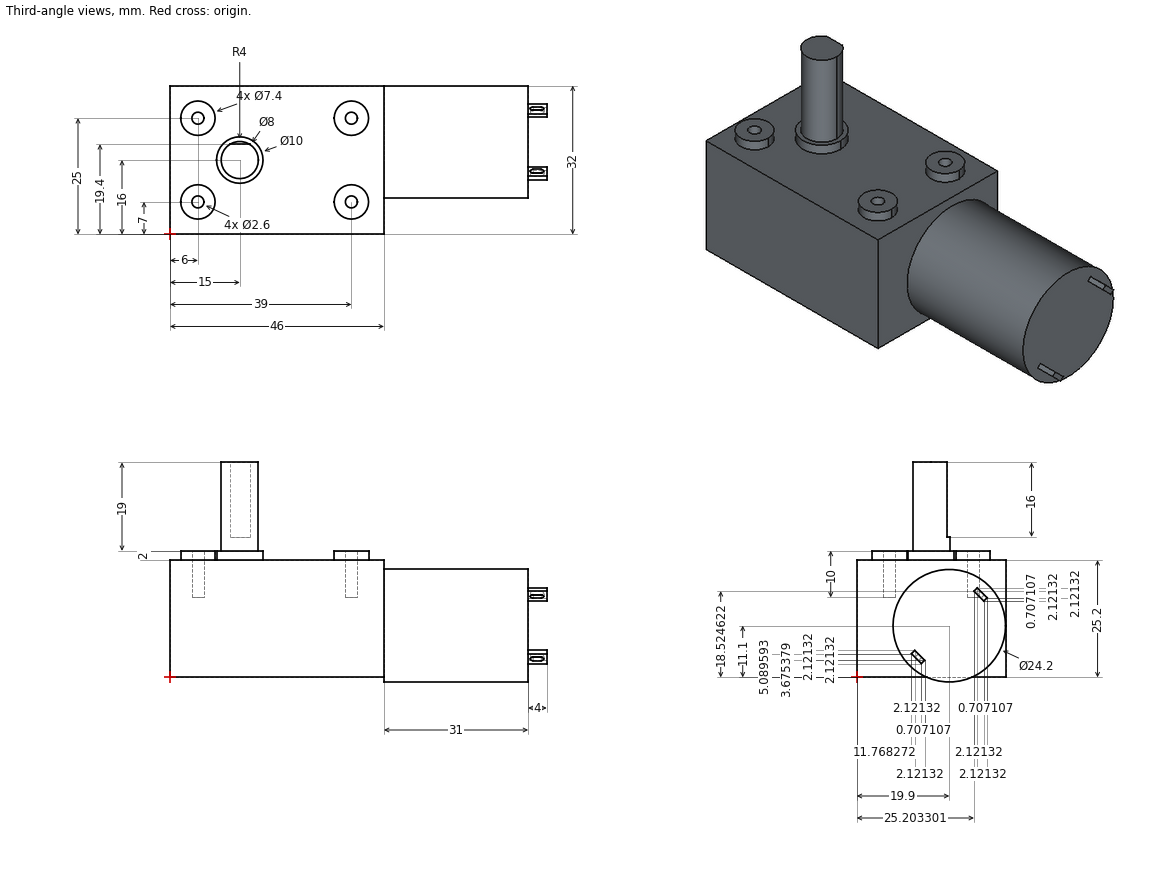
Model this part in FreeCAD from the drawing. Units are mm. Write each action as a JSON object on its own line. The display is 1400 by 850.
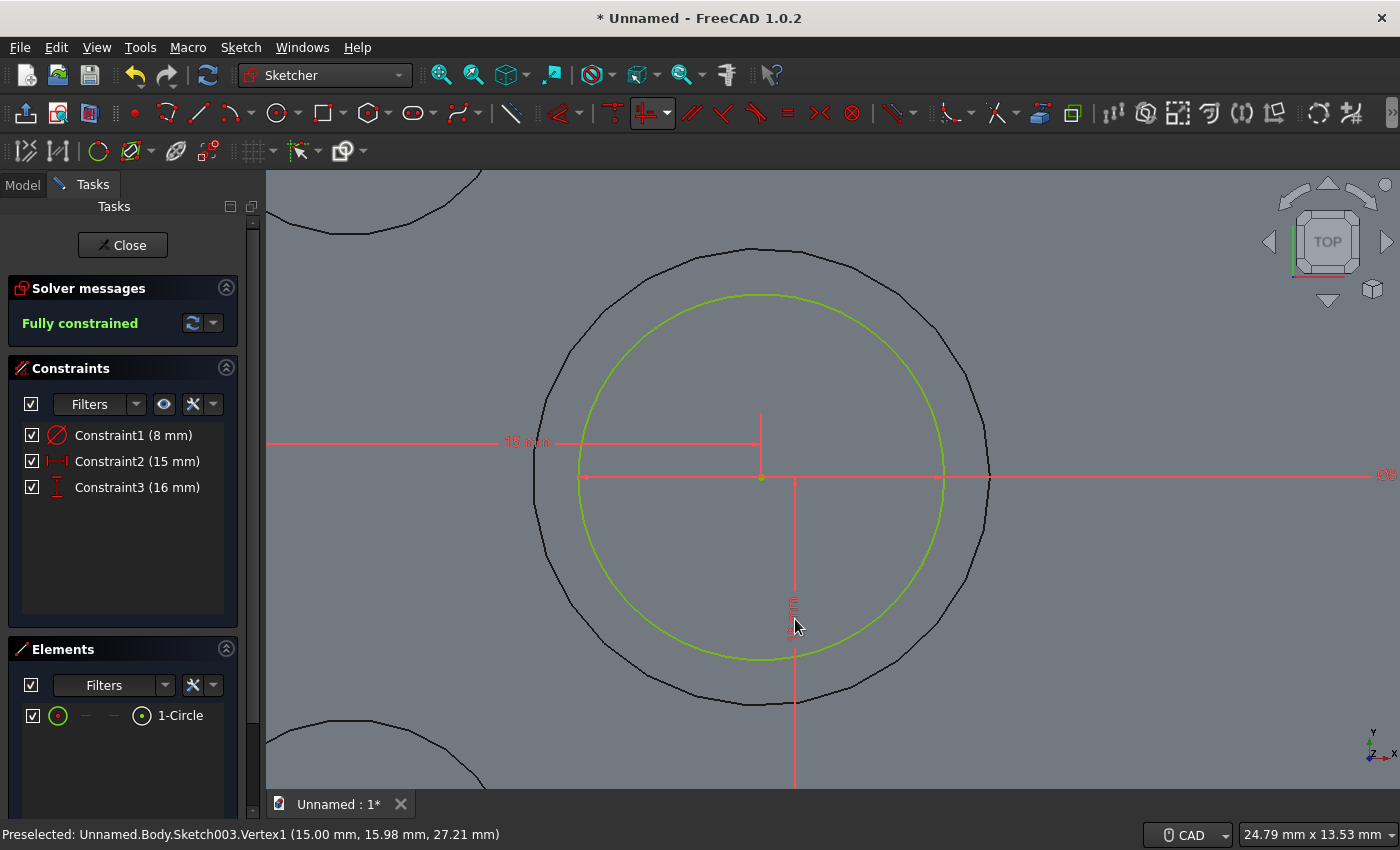
{"action": "left_click", "coordinate": [123, 245]}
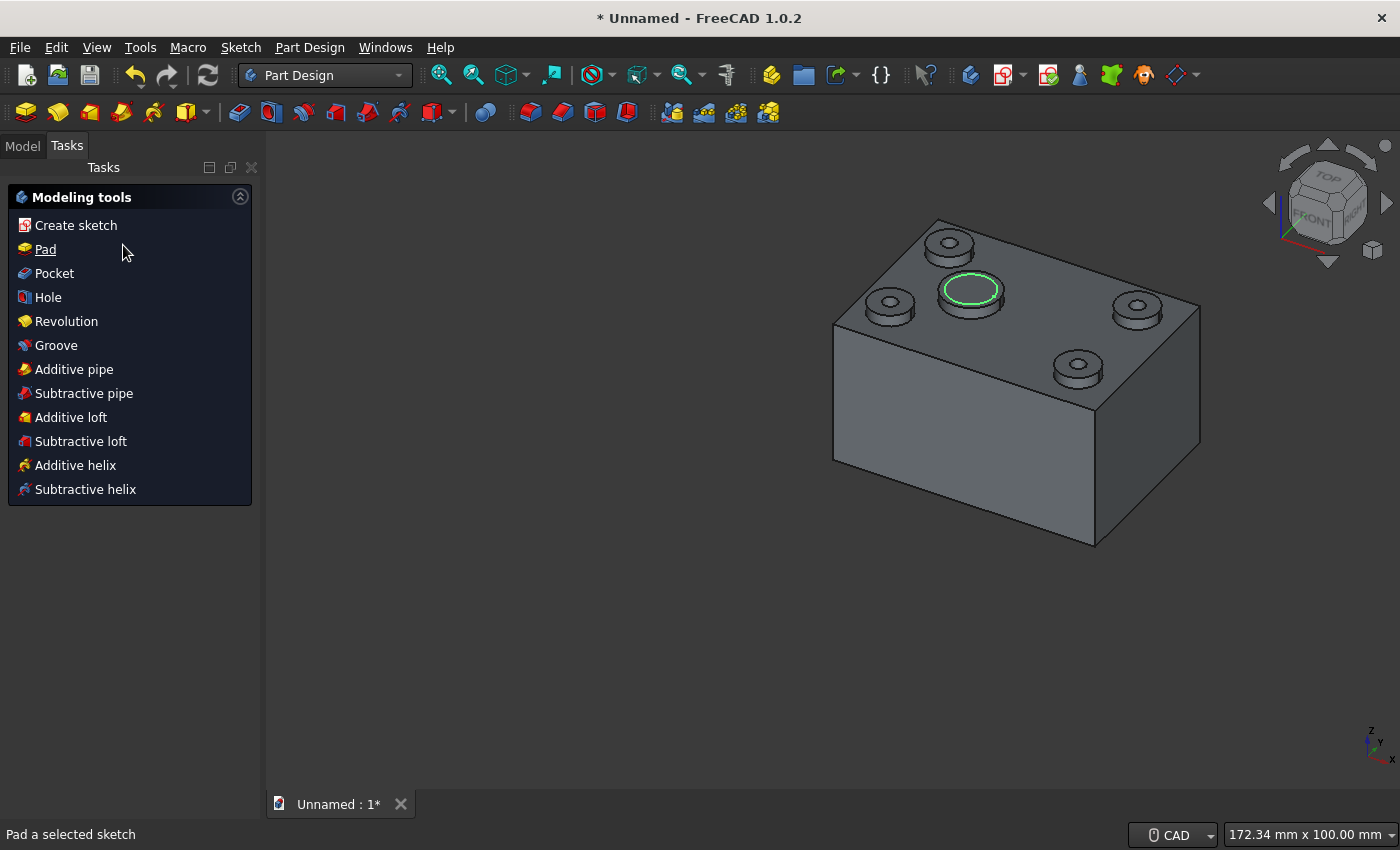
{"action": "left_click", "coordinate": [26, 112]}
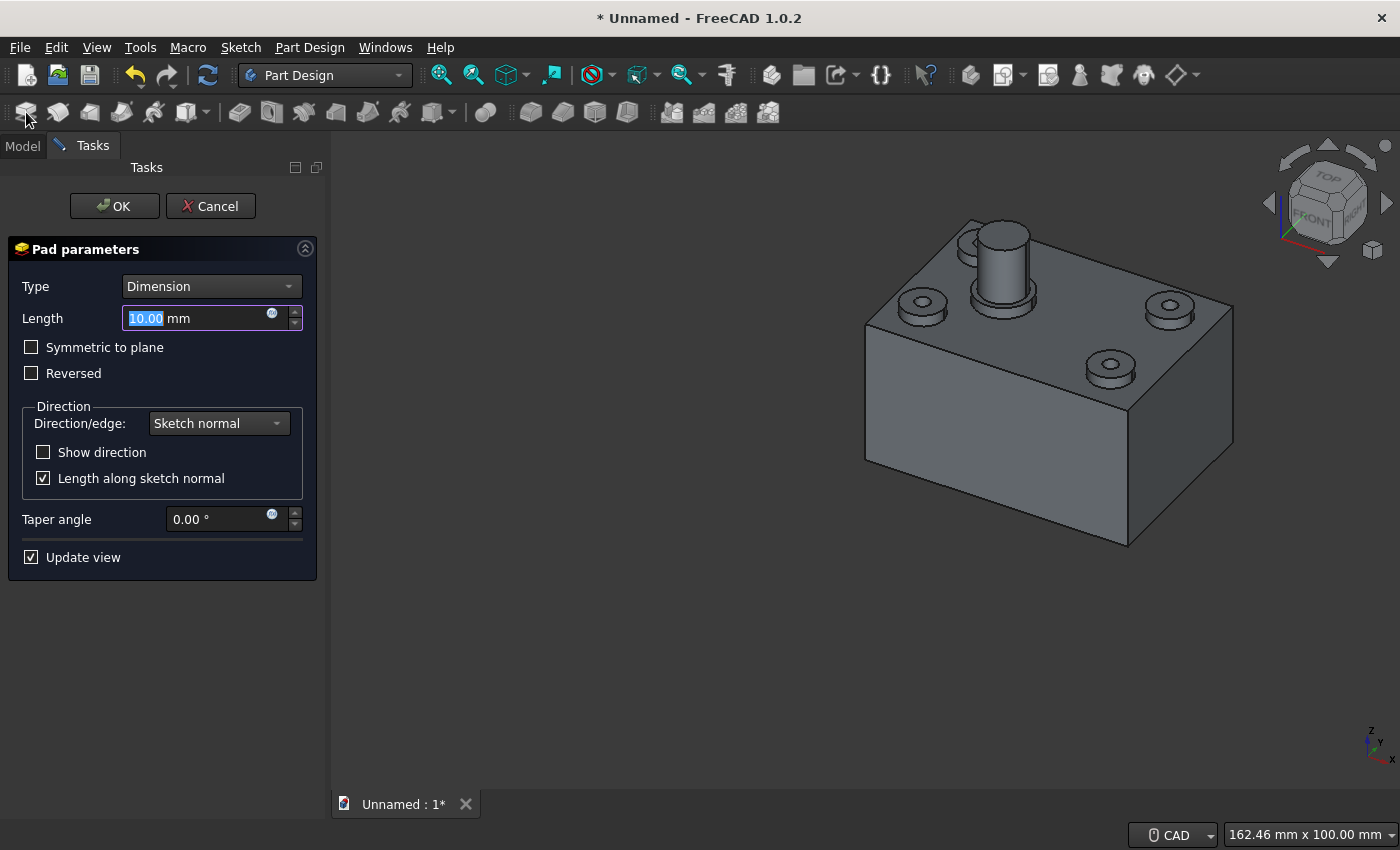
{"action": "type", "text": "19"}
{"action": "key", "text": "Tab"}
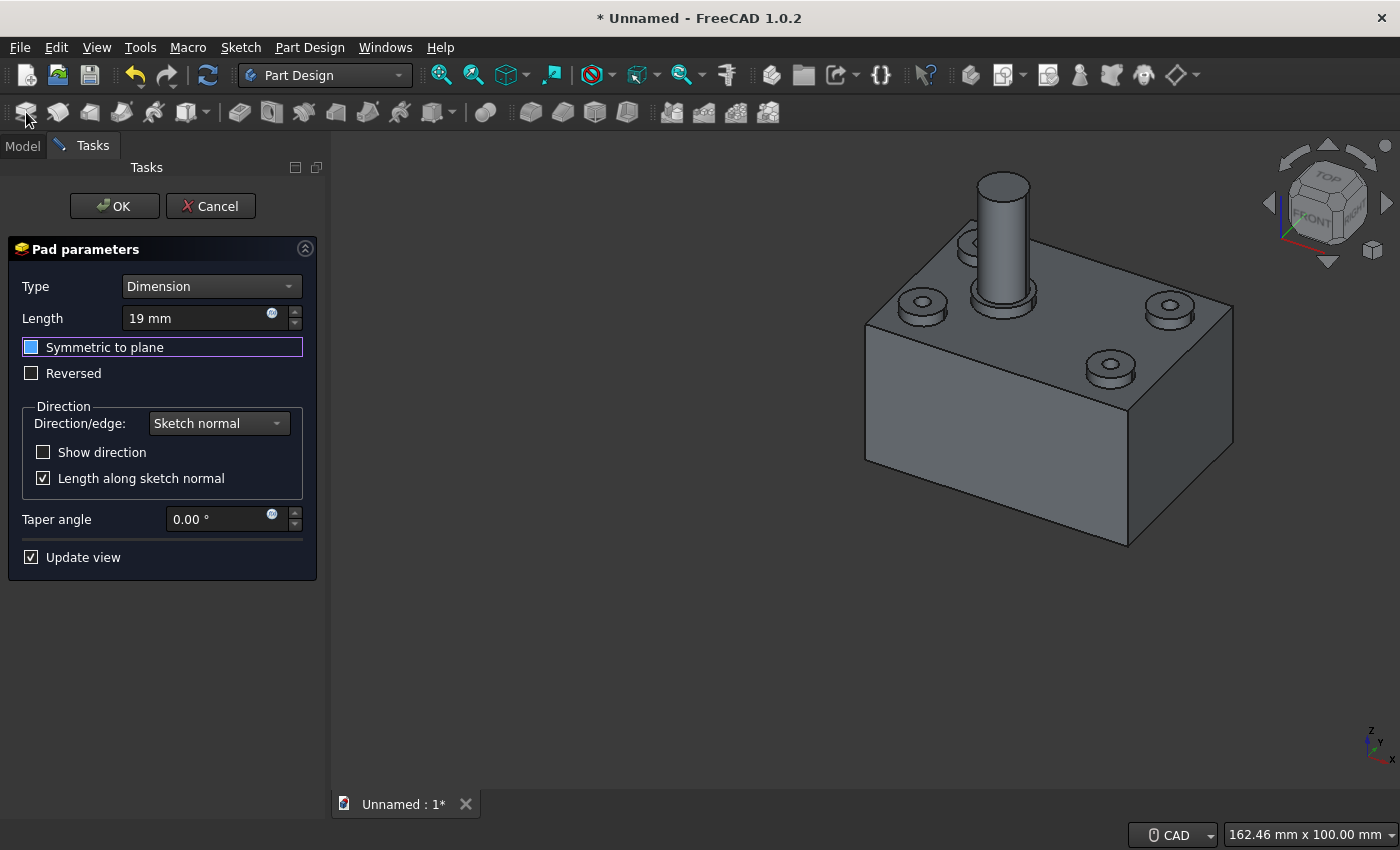
{"action": "left_click", "coordinate": [115, 206]}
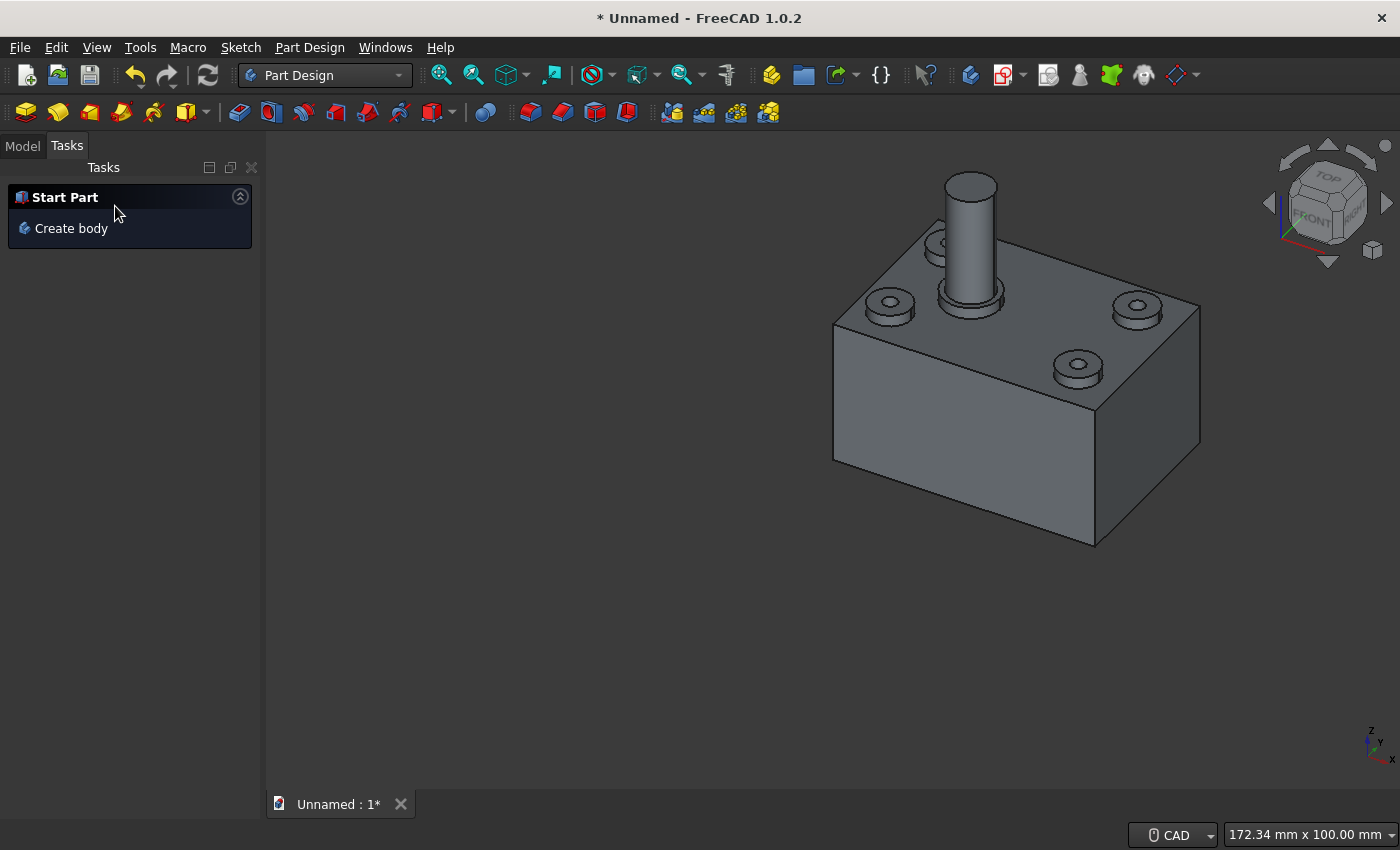
{"action": "left_click", "coordinate": [442, 76]}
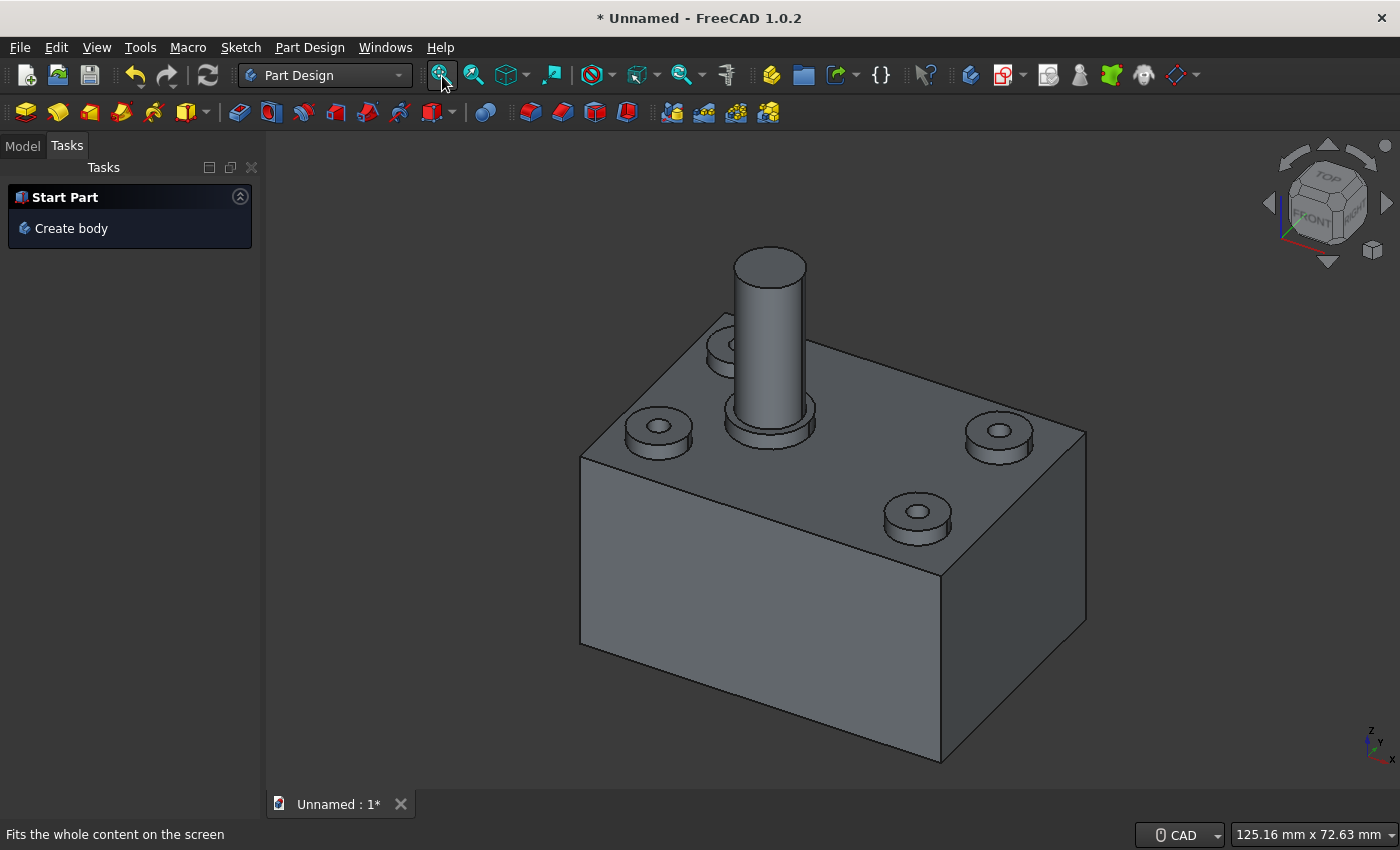
{"action": "left_click", "coordinate": [23, 145]}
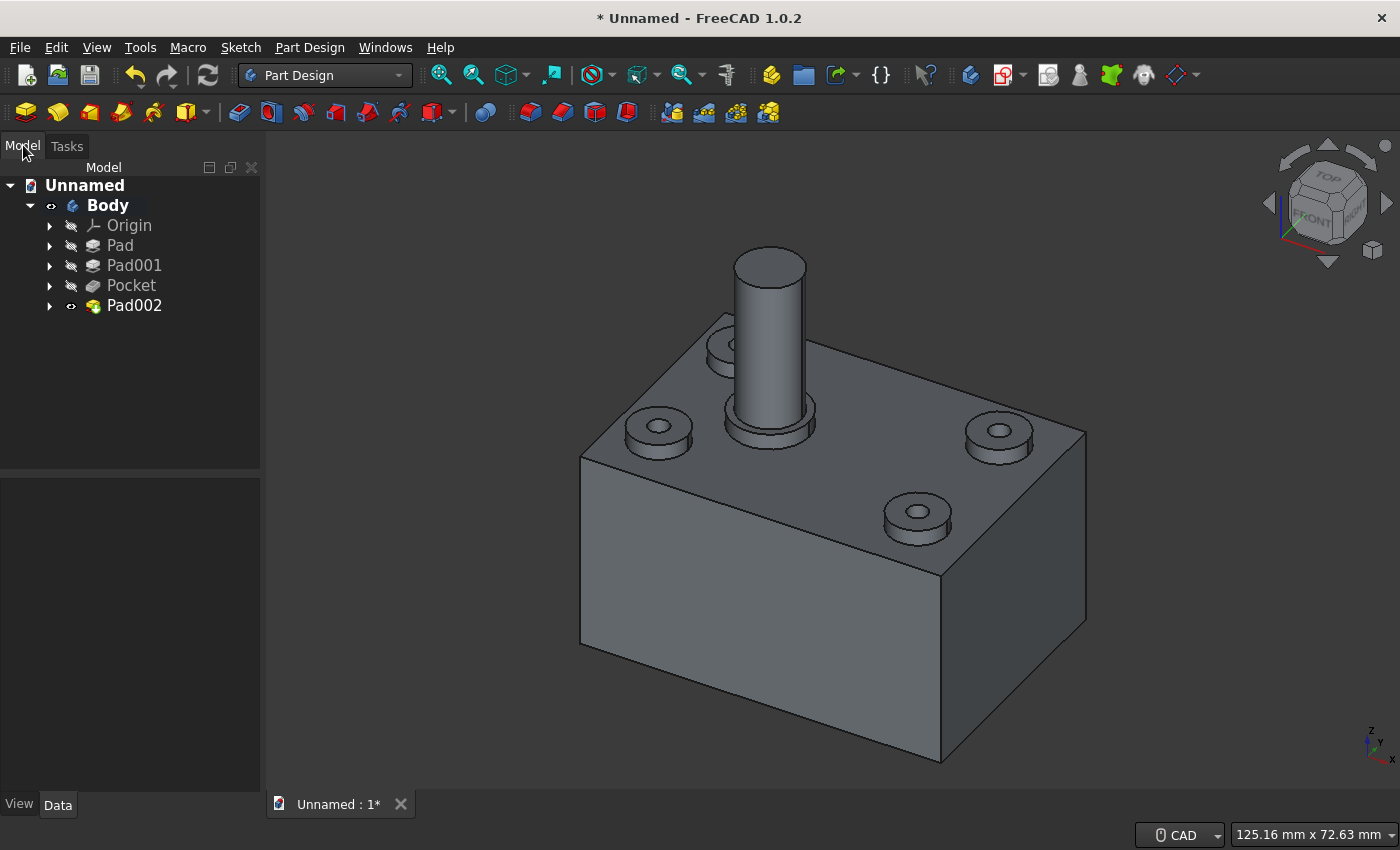
{"action": "left_click", "coordinate": [50, 226]}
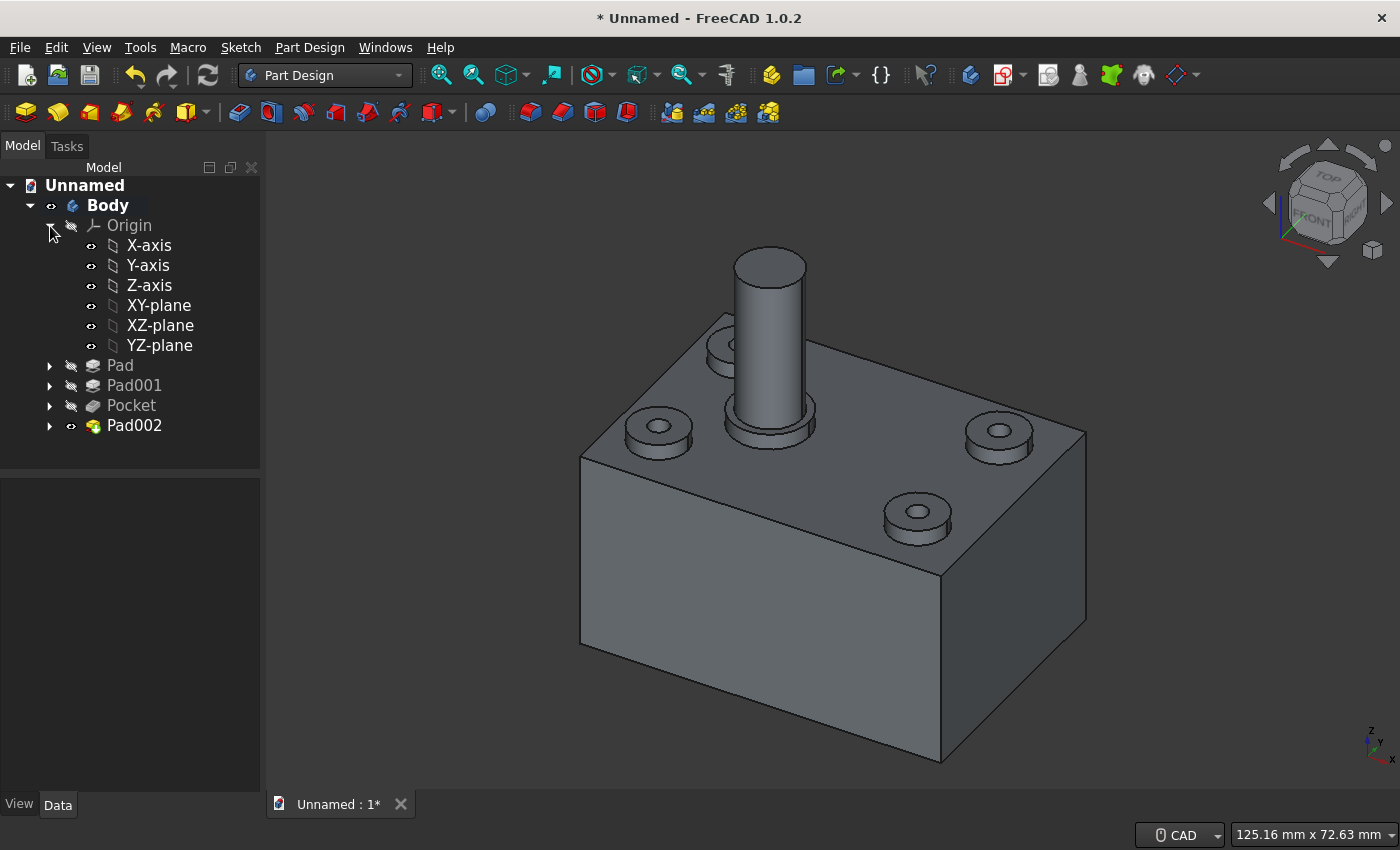
{"action": "left_click", "coordinate": [136, 306]}